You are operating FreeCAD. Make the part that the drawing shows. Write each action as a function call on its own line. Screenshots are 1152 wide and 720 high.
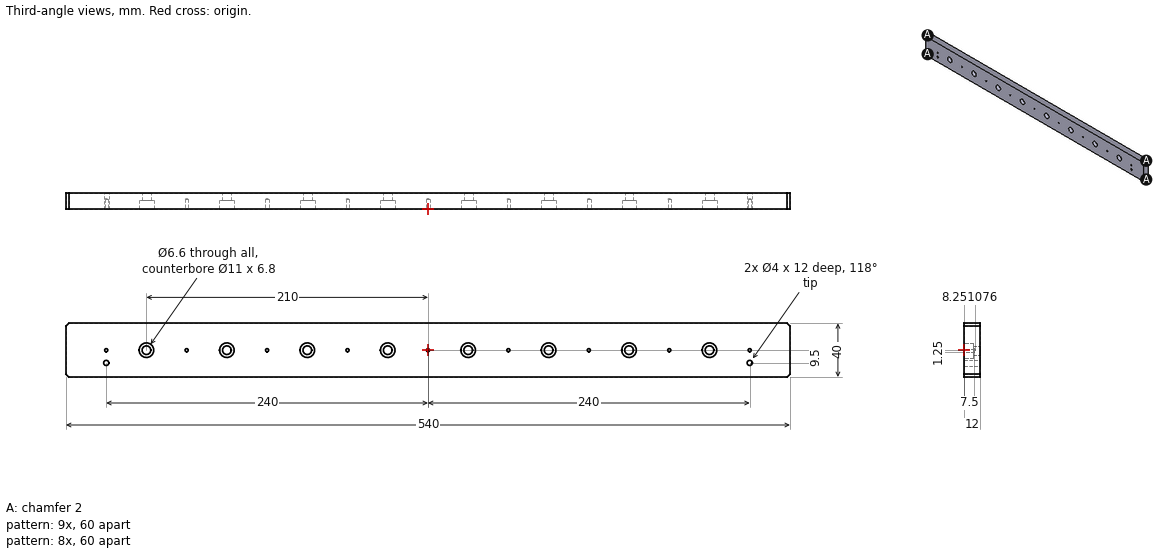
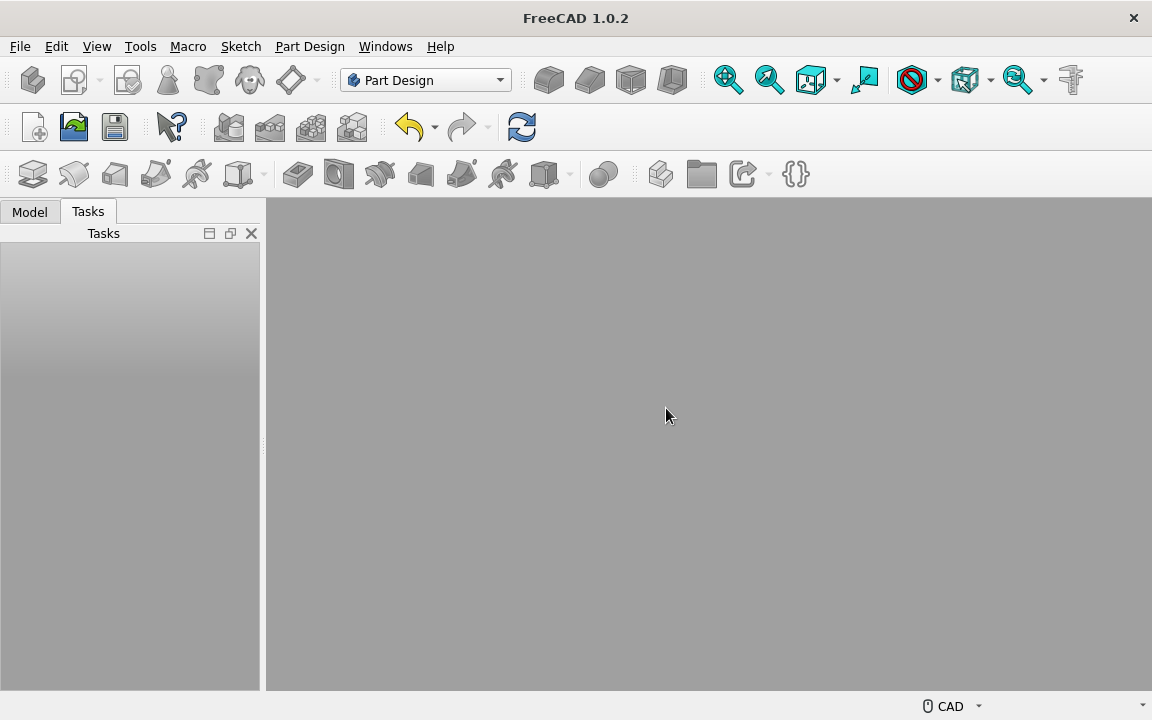
click(33, 128)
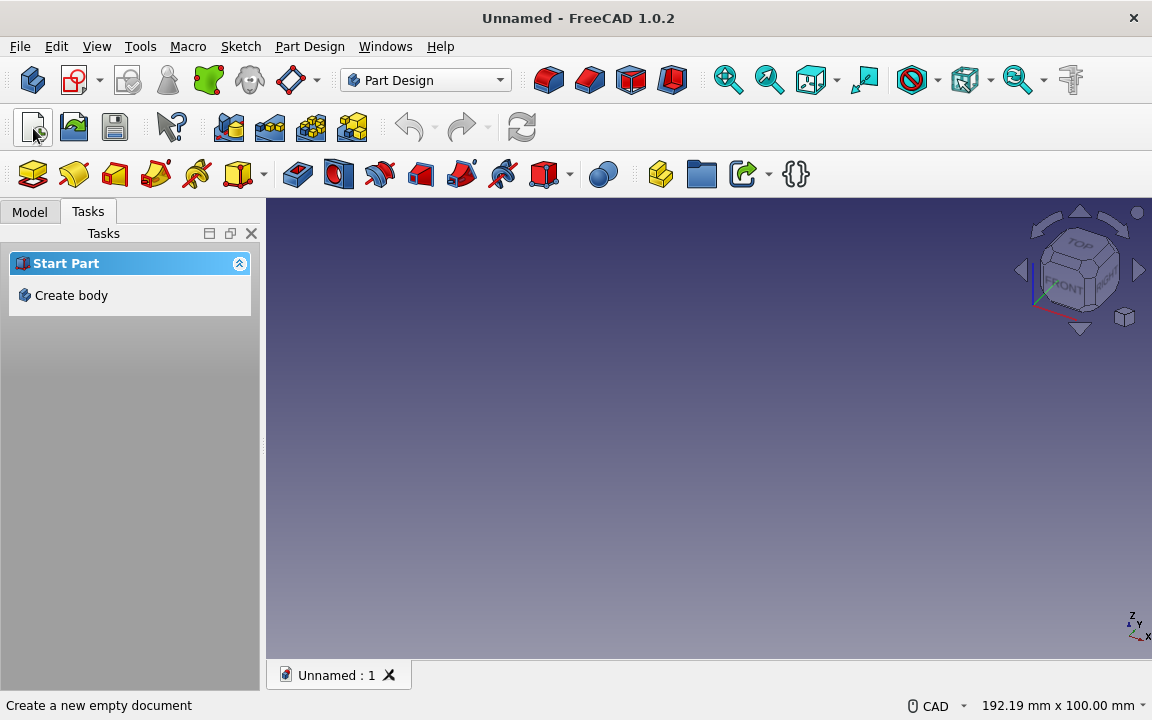
click(74, 80)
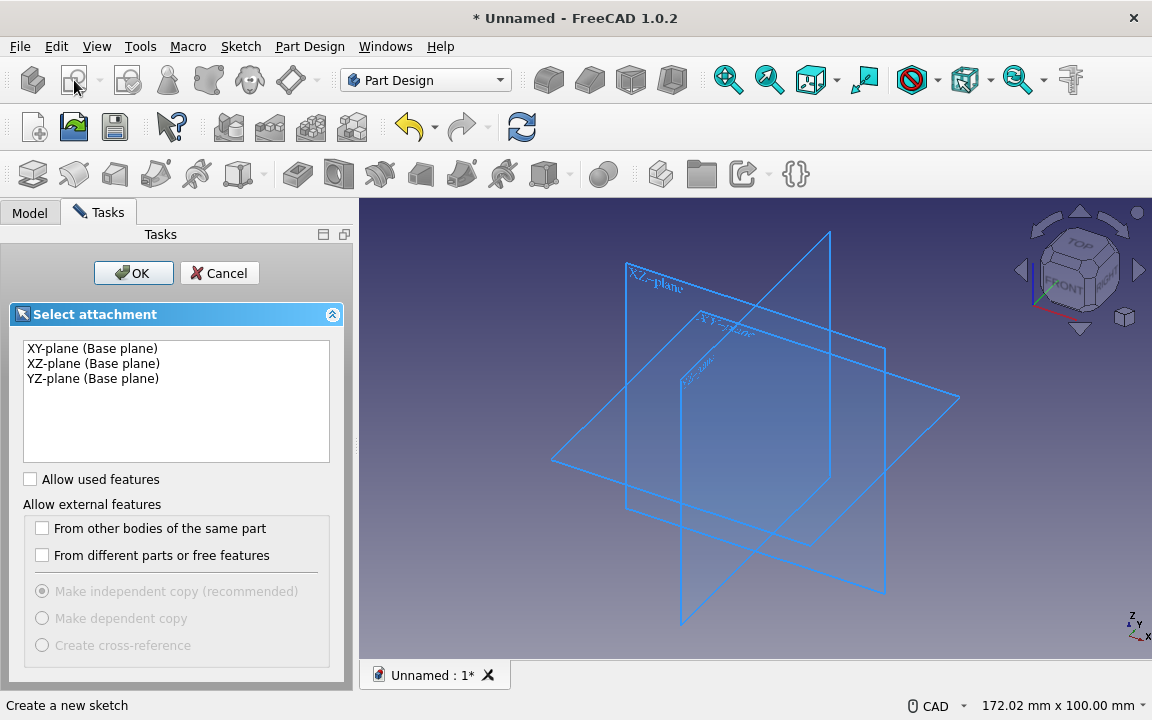
click(84, 364)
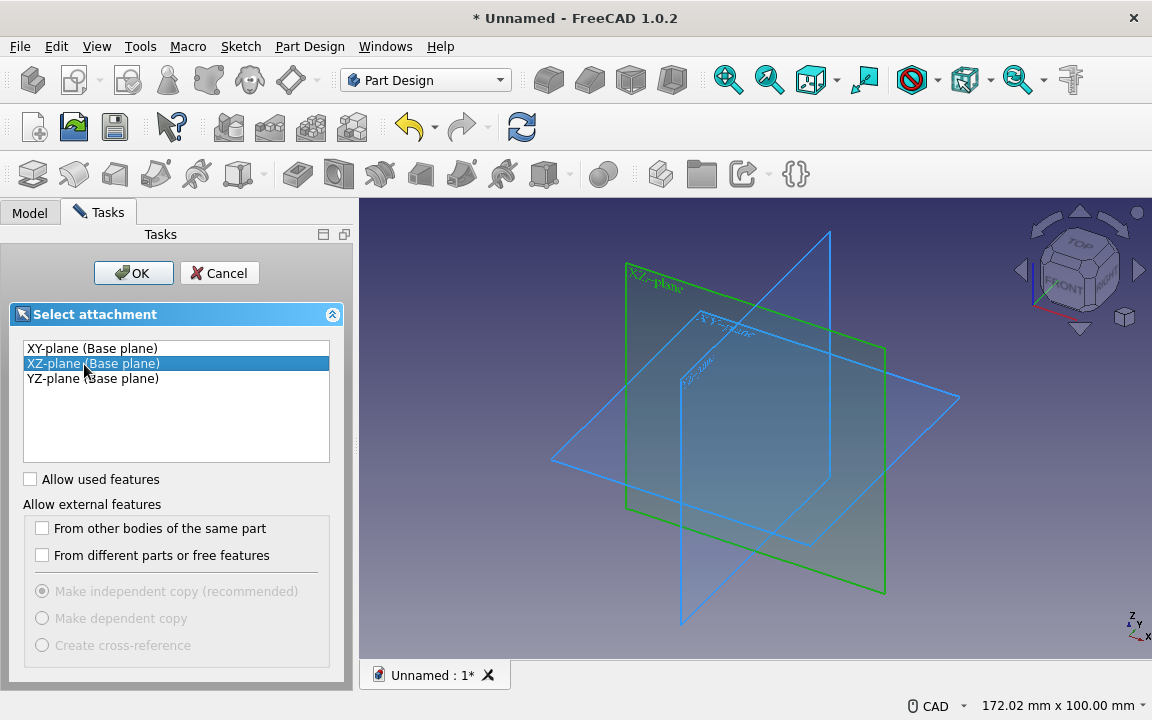
click(134, 273)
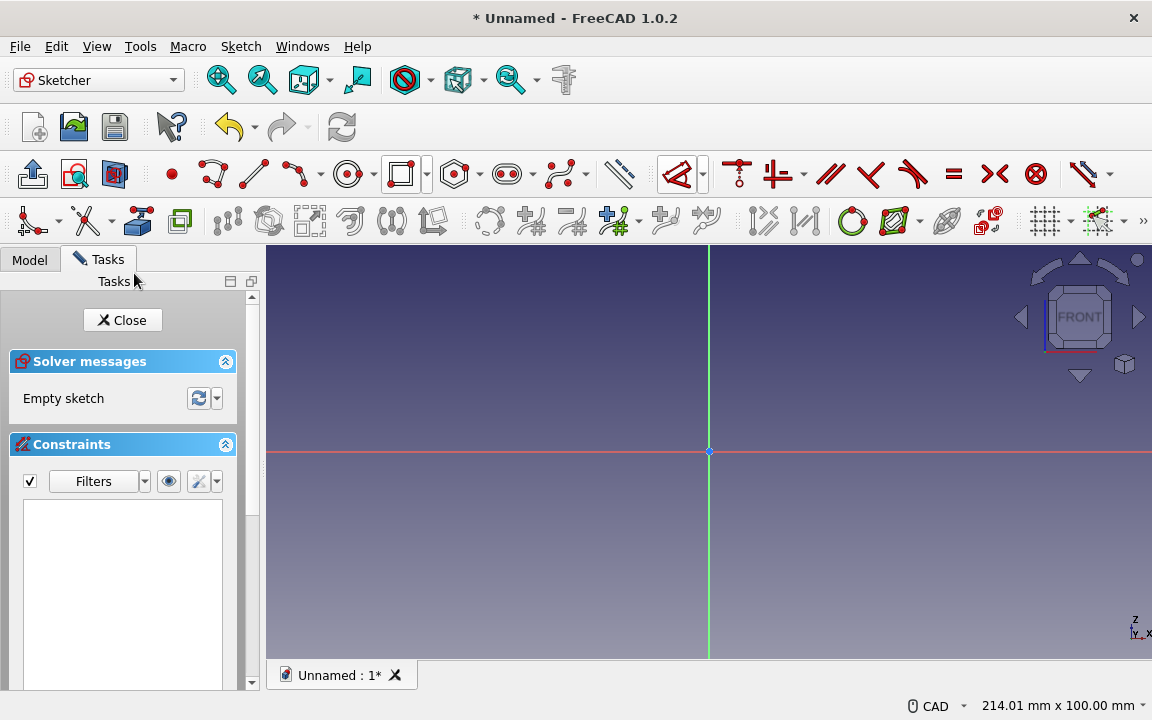
scroll(623, 452, down, 8)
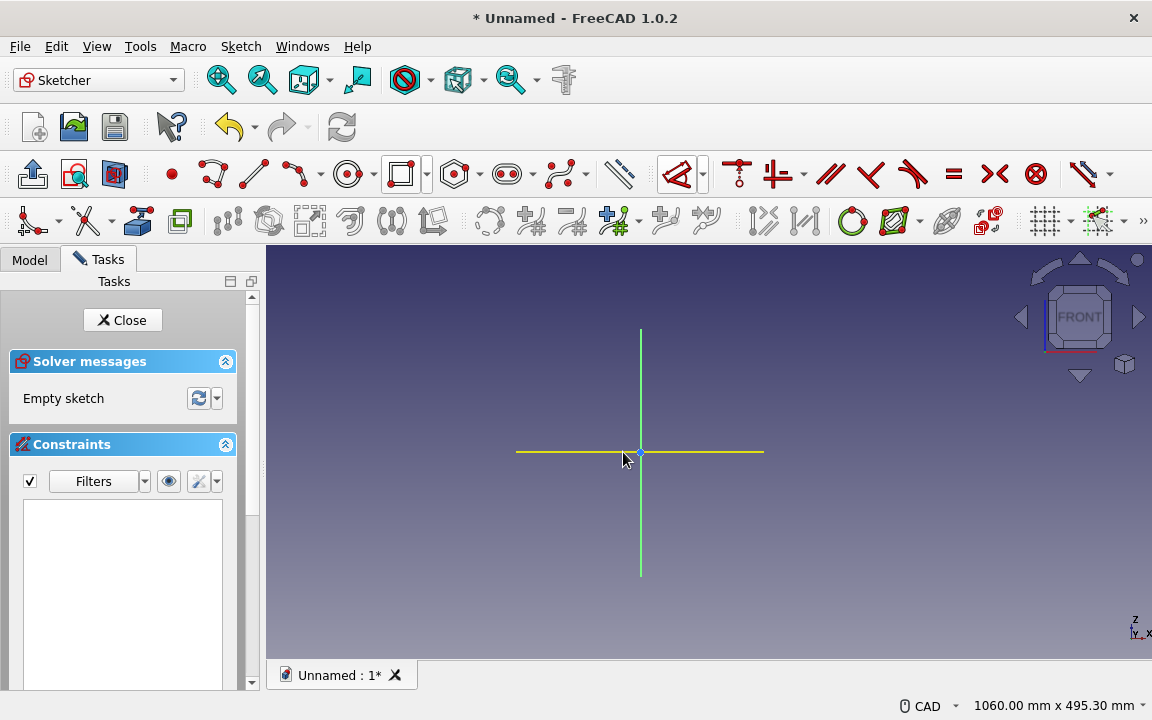
key(g)
key(v)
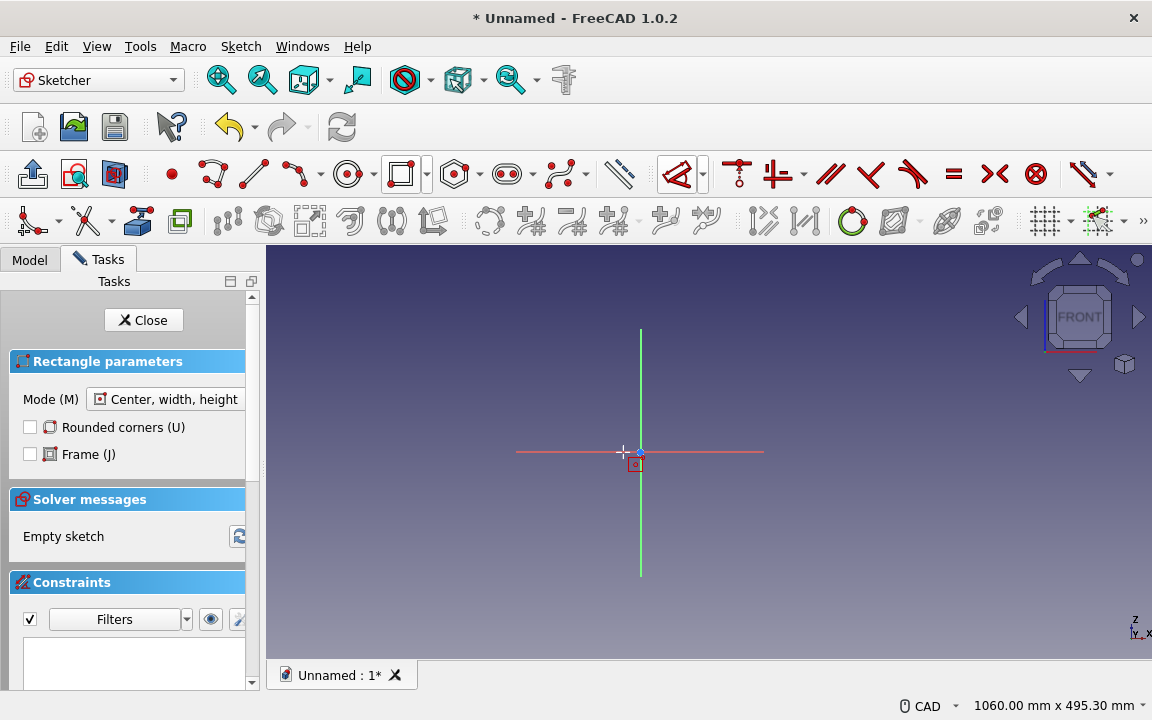
click(641, 452)
click(866, 436)
key(Escape)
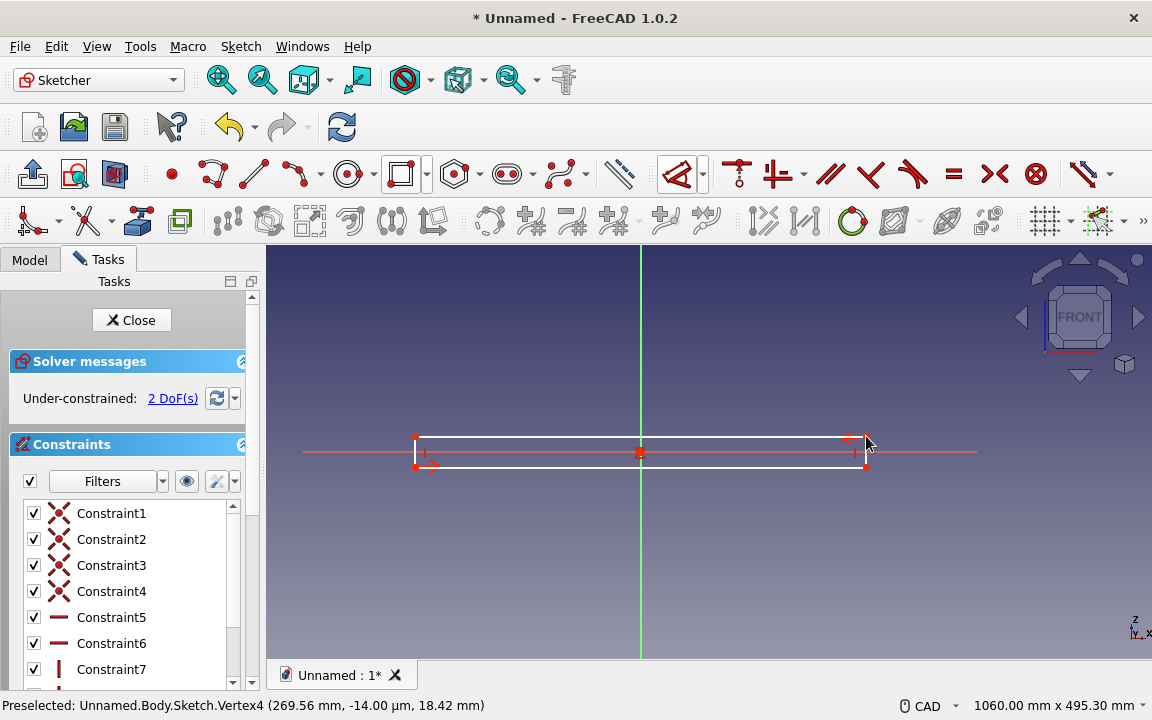
click(676, 174)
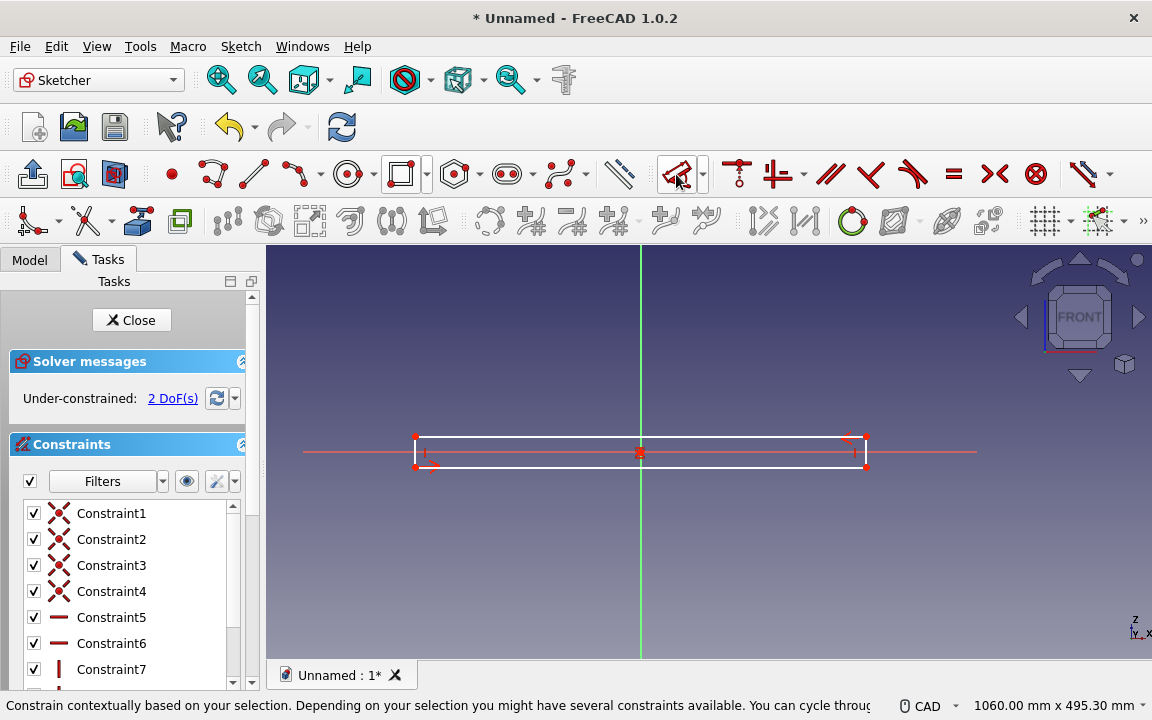
click(866, 455)
click(900, 445)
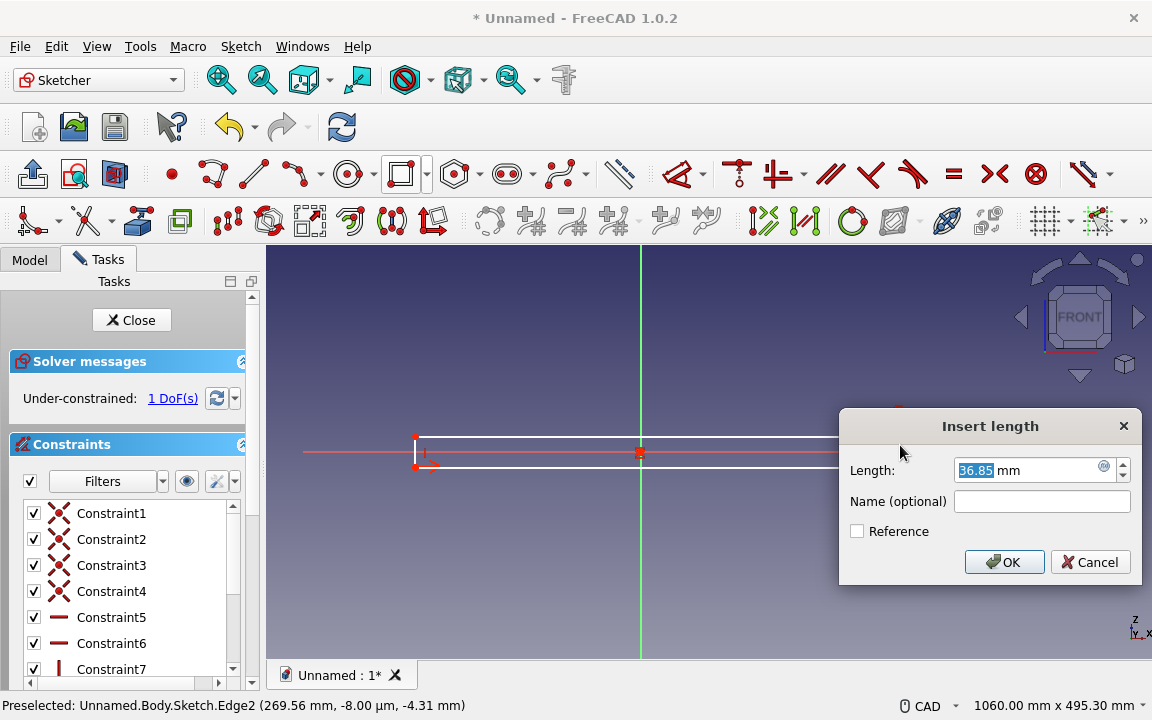
text(40)
key(Return)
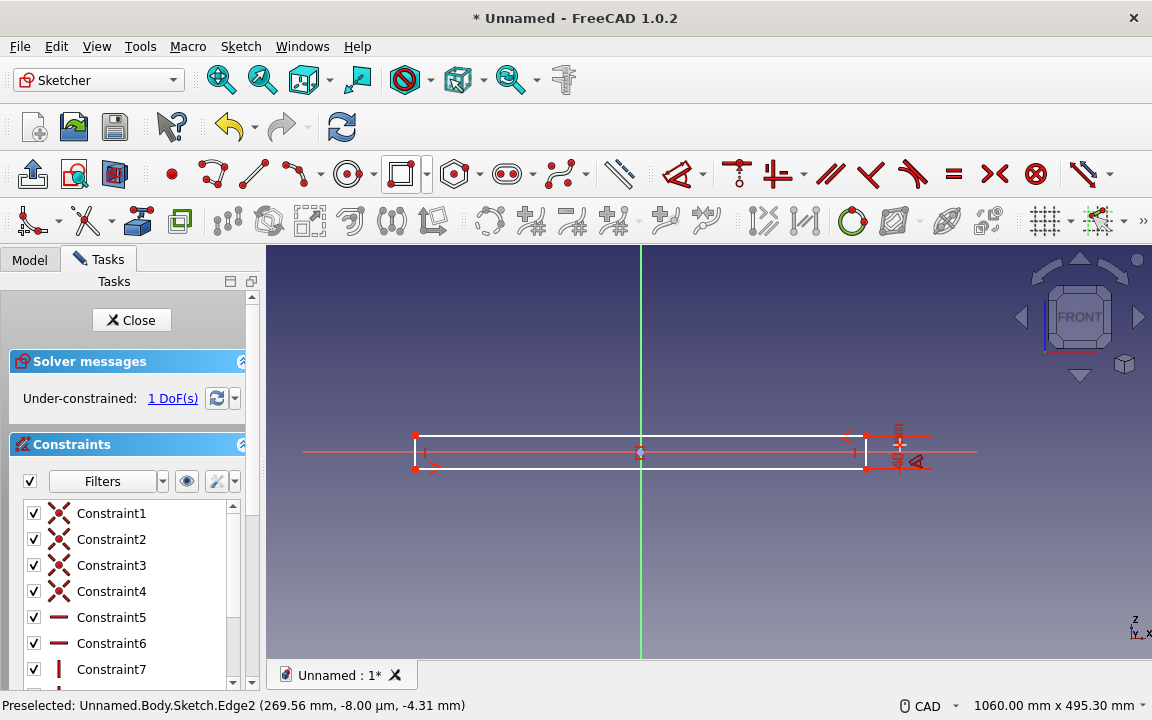
click(551, 469)
click(537, 503)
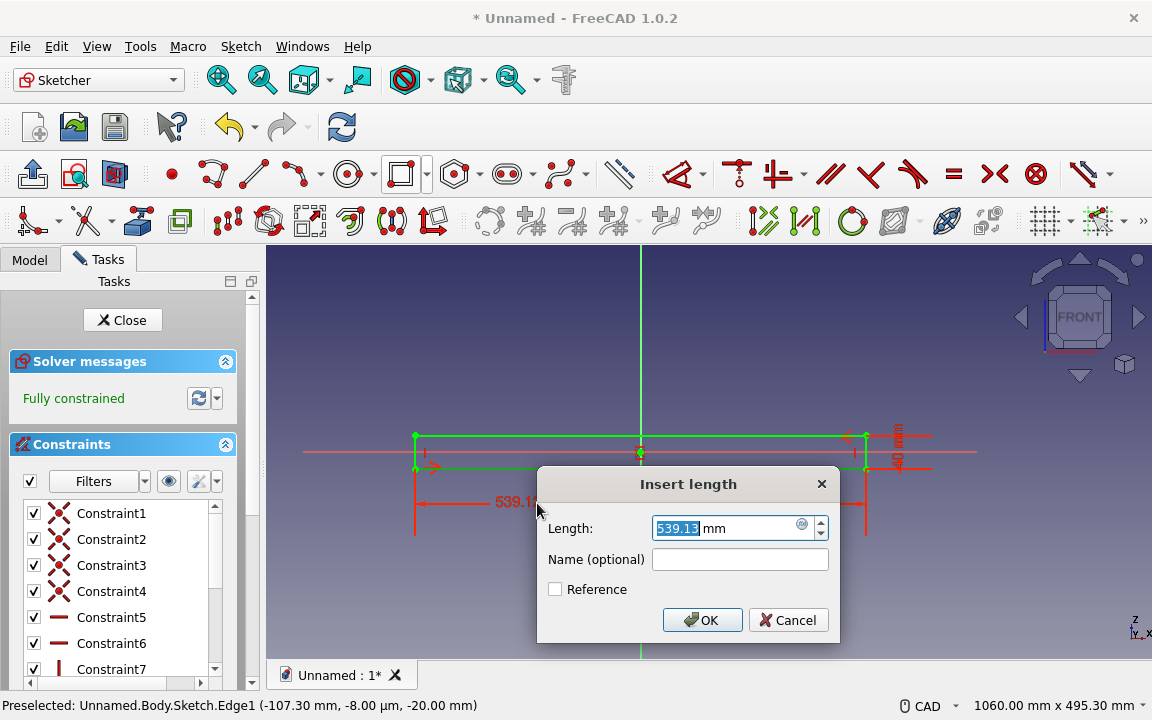
text(540)
key(Return)
key(Escape)